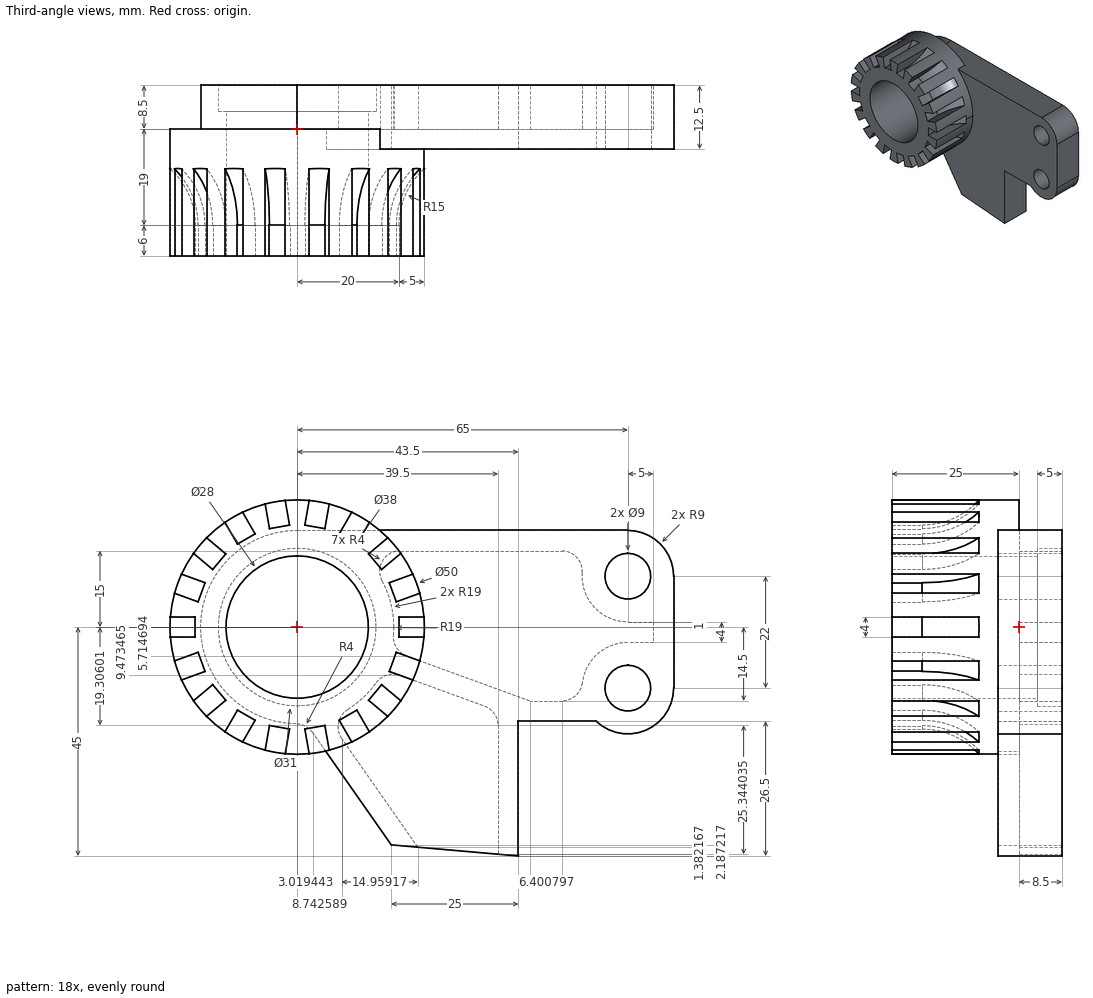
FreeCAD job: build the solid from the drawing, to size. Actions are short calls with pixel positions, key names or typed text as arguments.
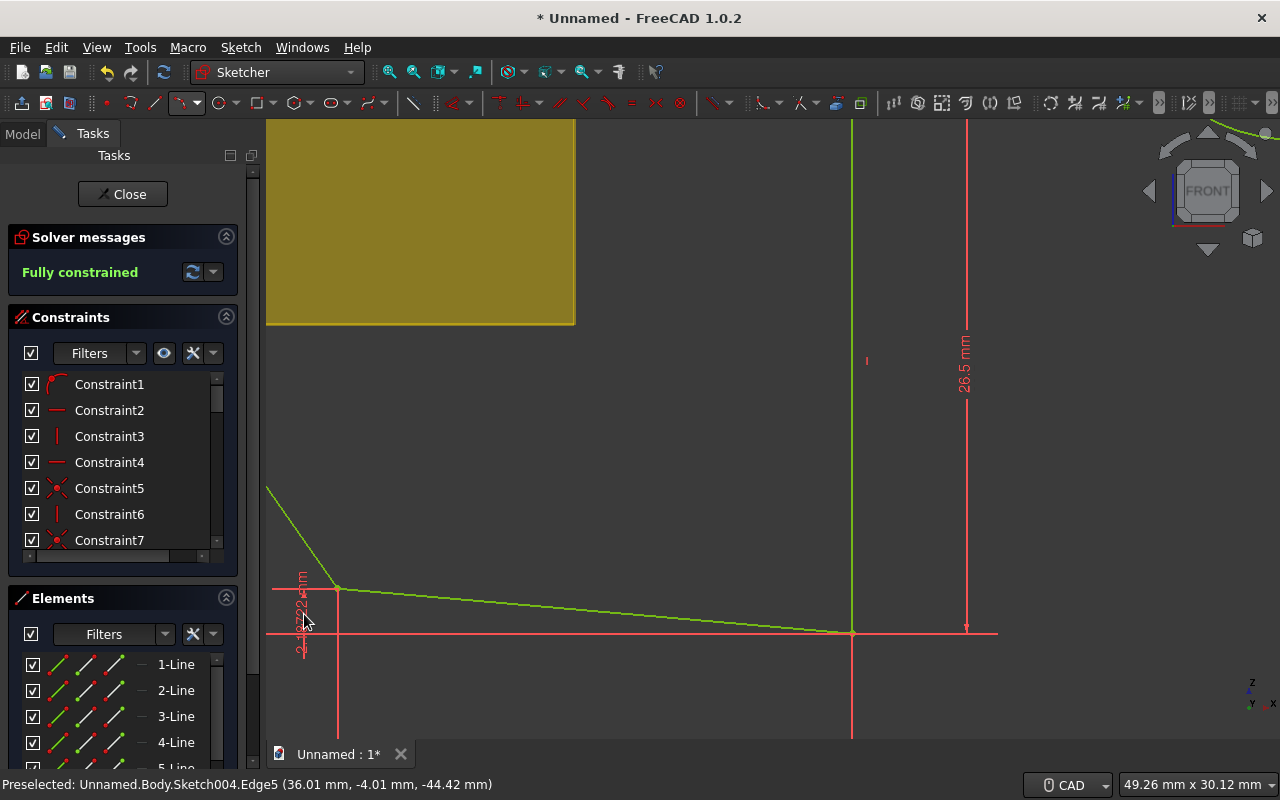
click(123, 194)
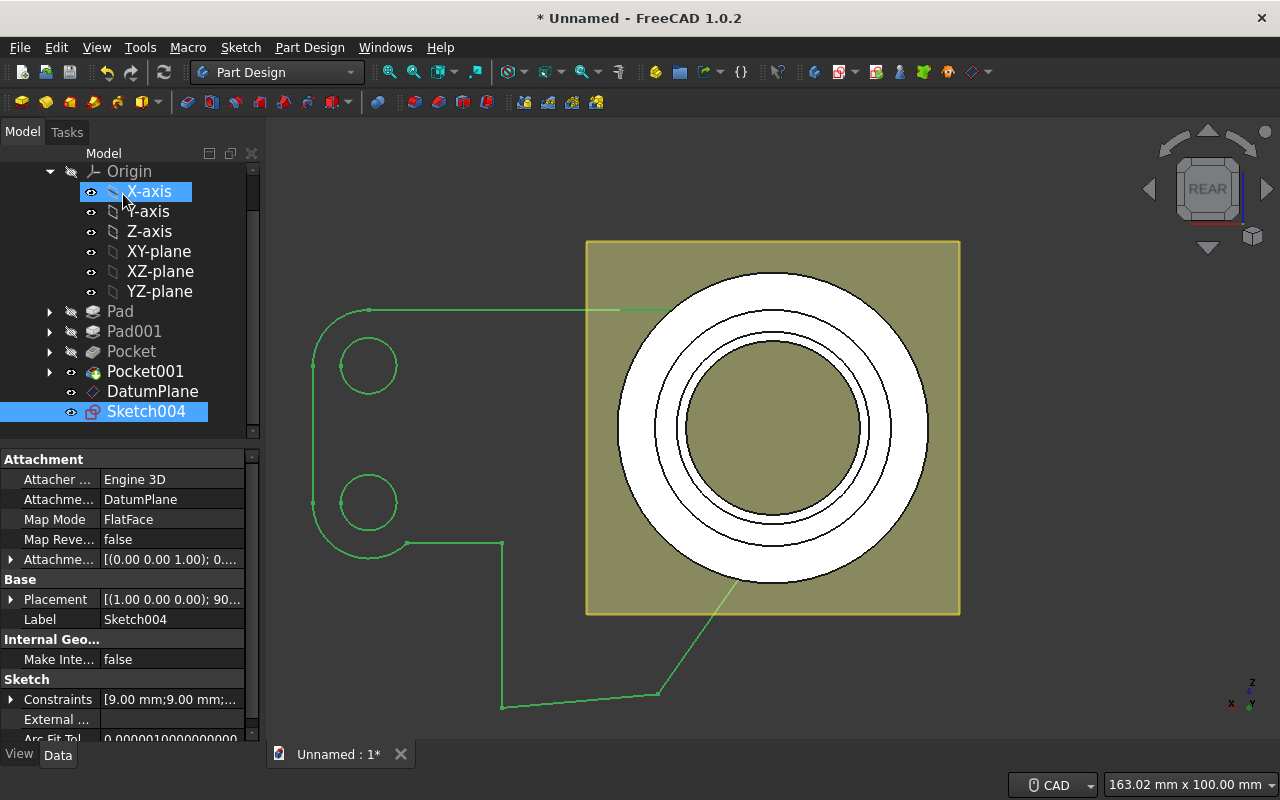
click(22, 102)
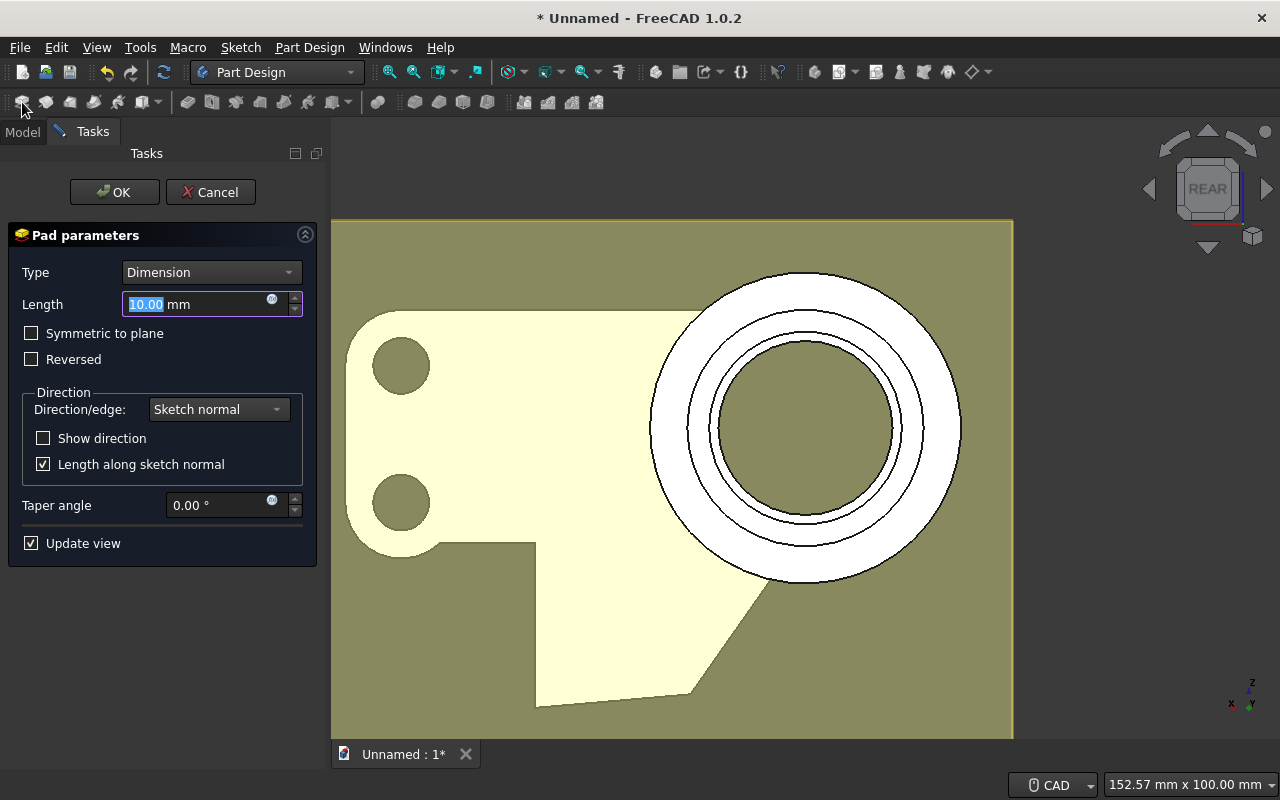
text(12.5)
key(Tab)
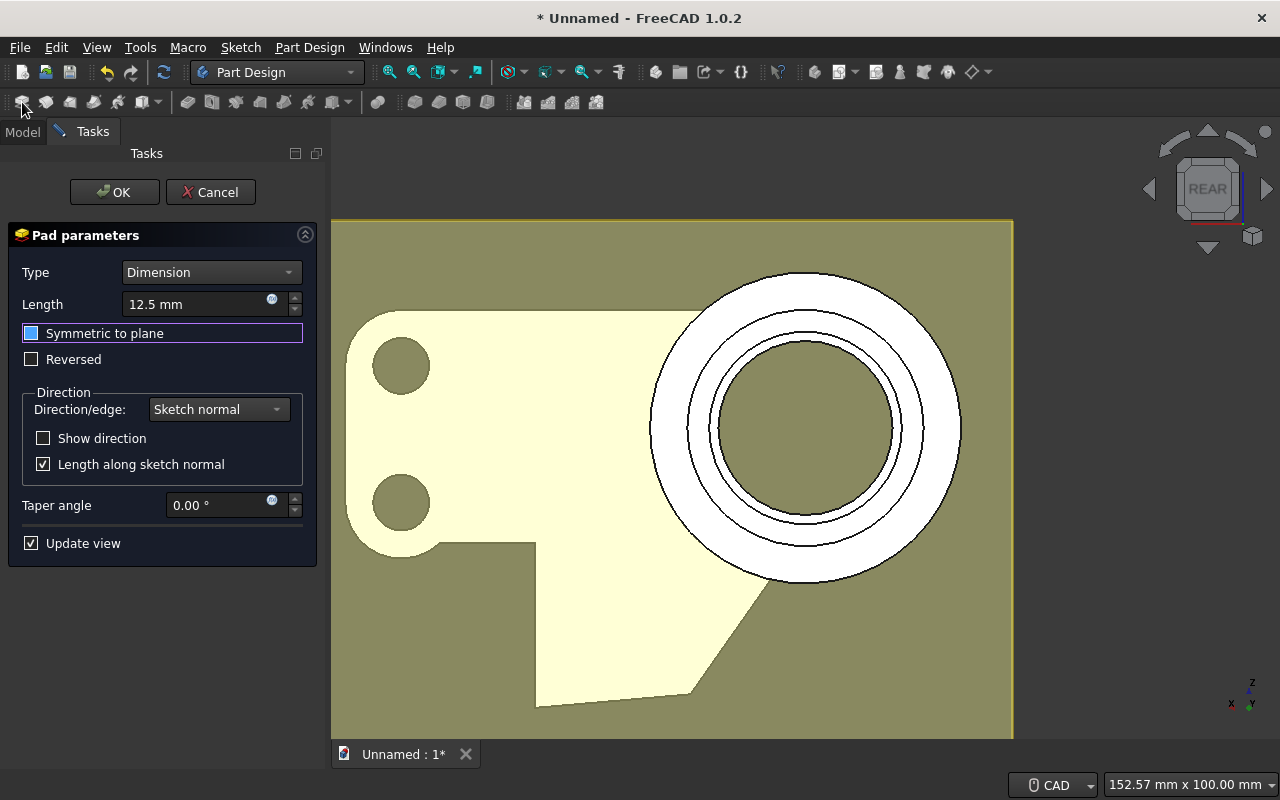
click(30, 359)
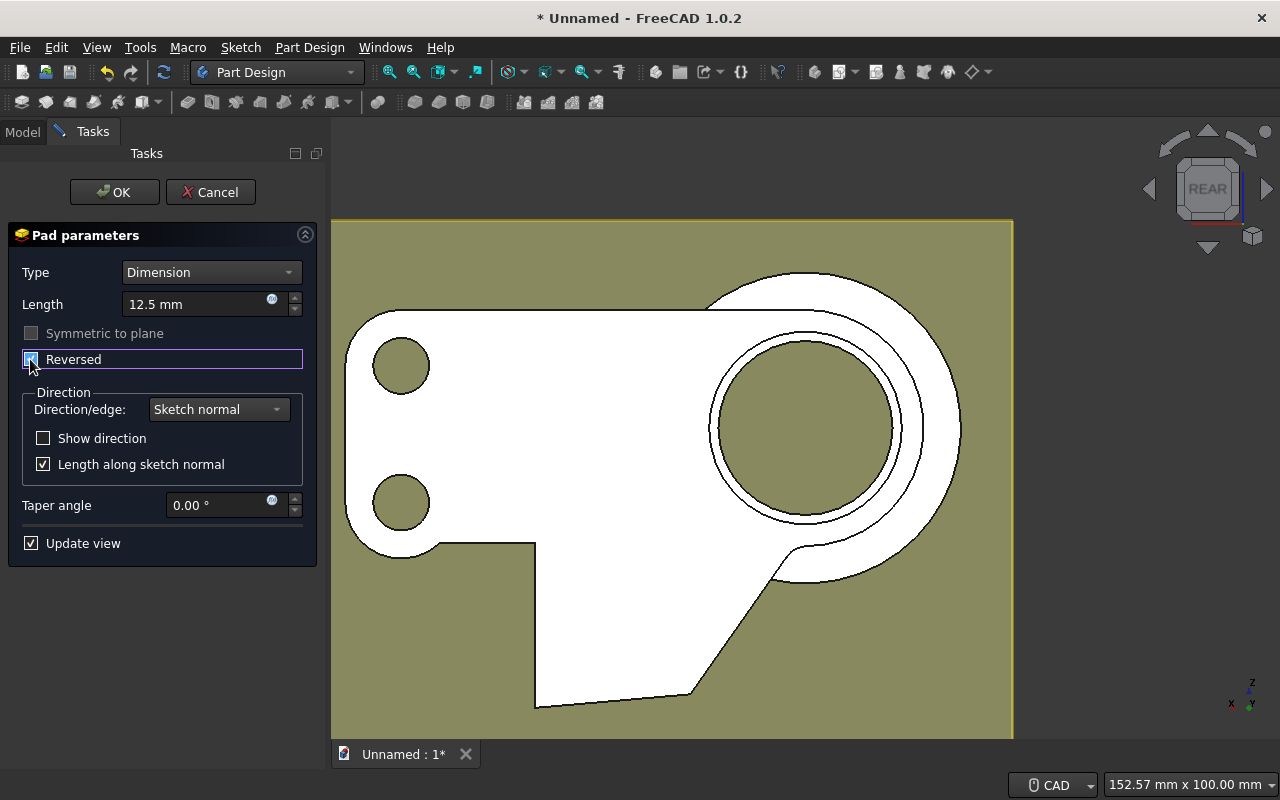
click(115, 192)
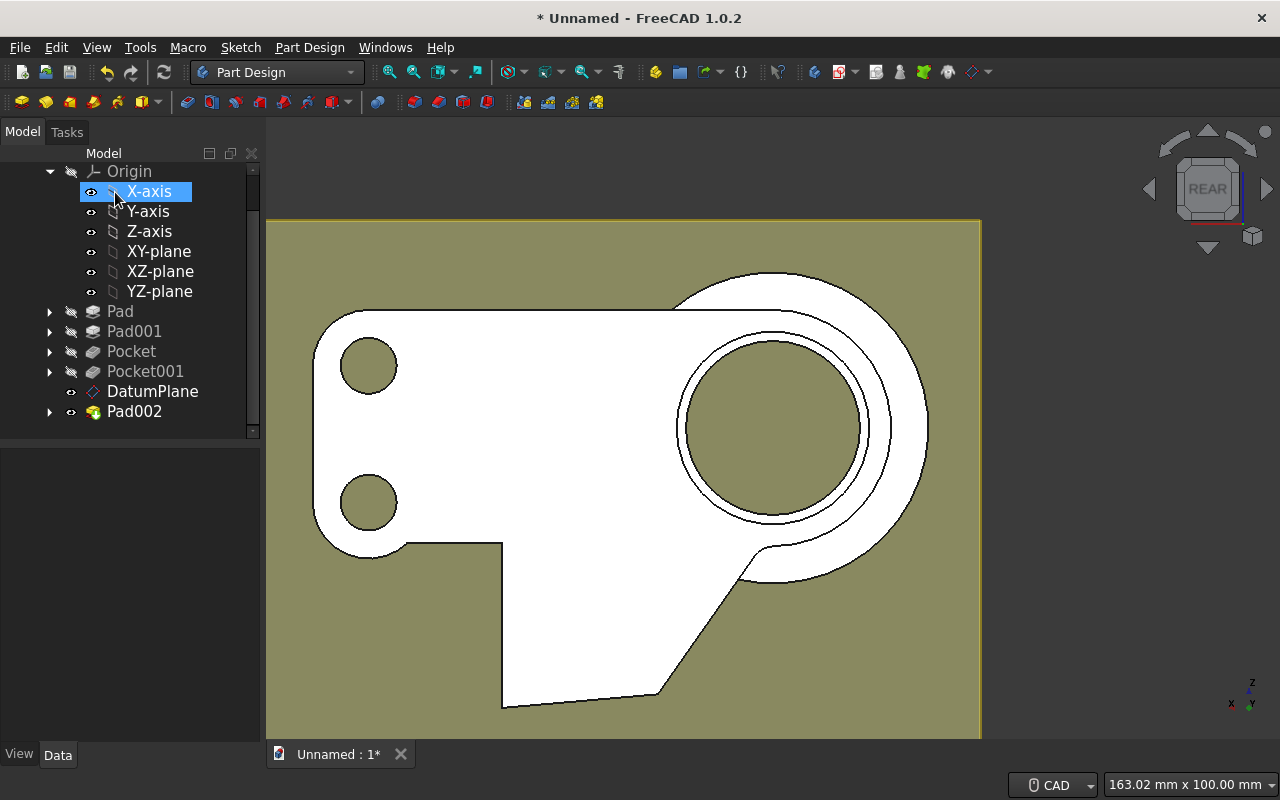
click(116, 392)
key(space)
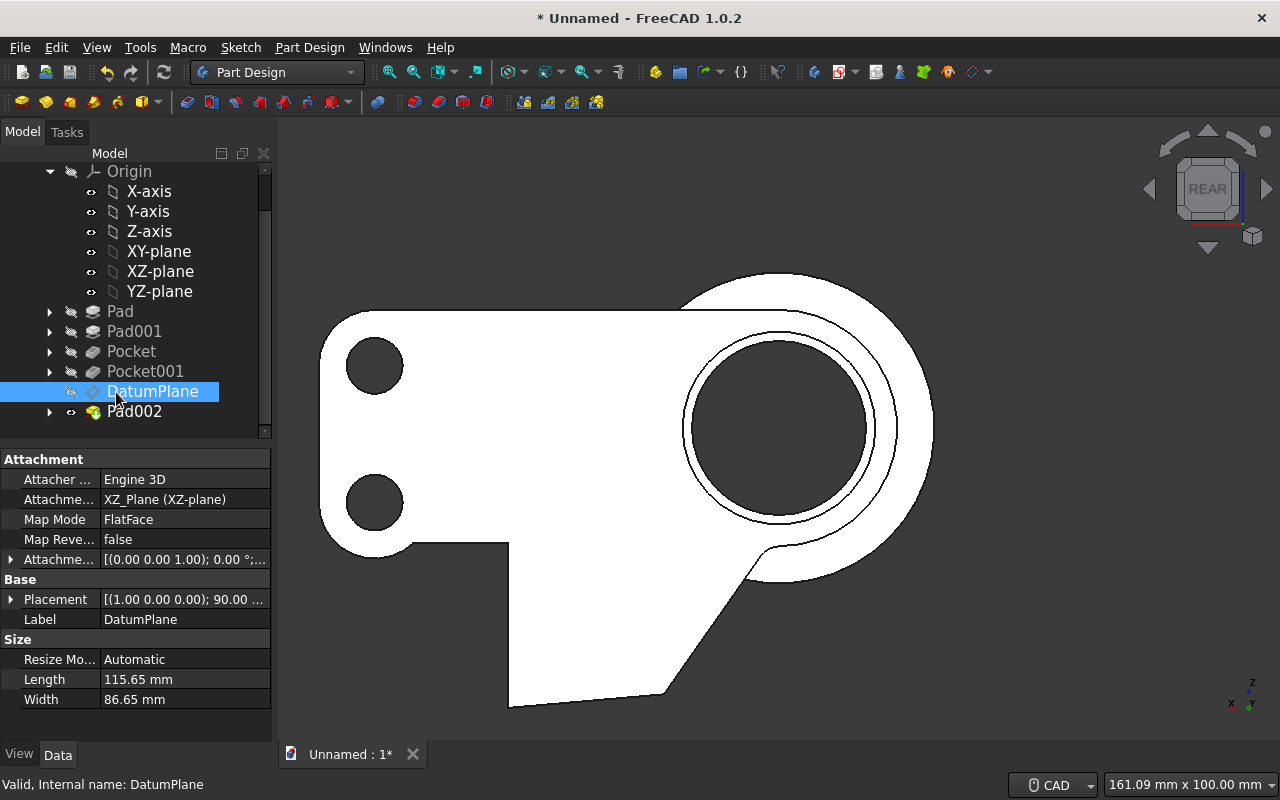
click(318, 699)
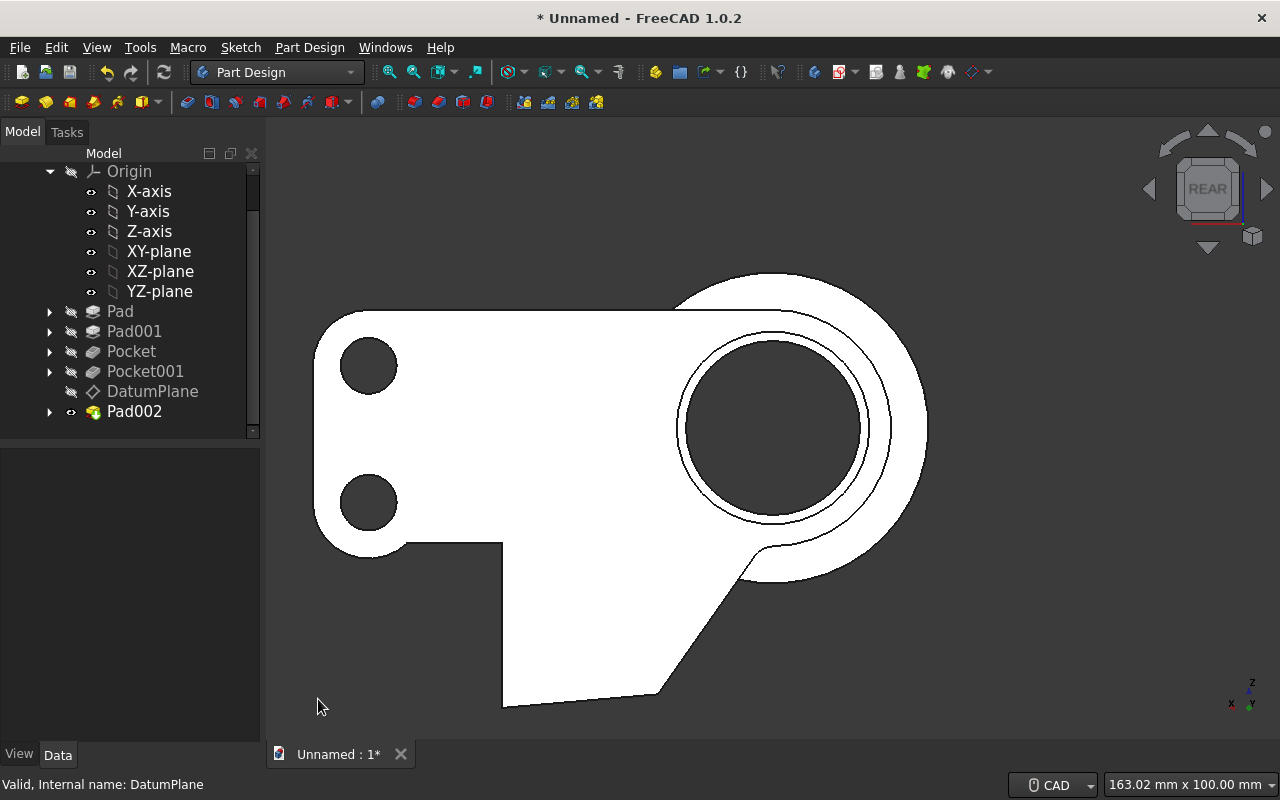
click(840, 72)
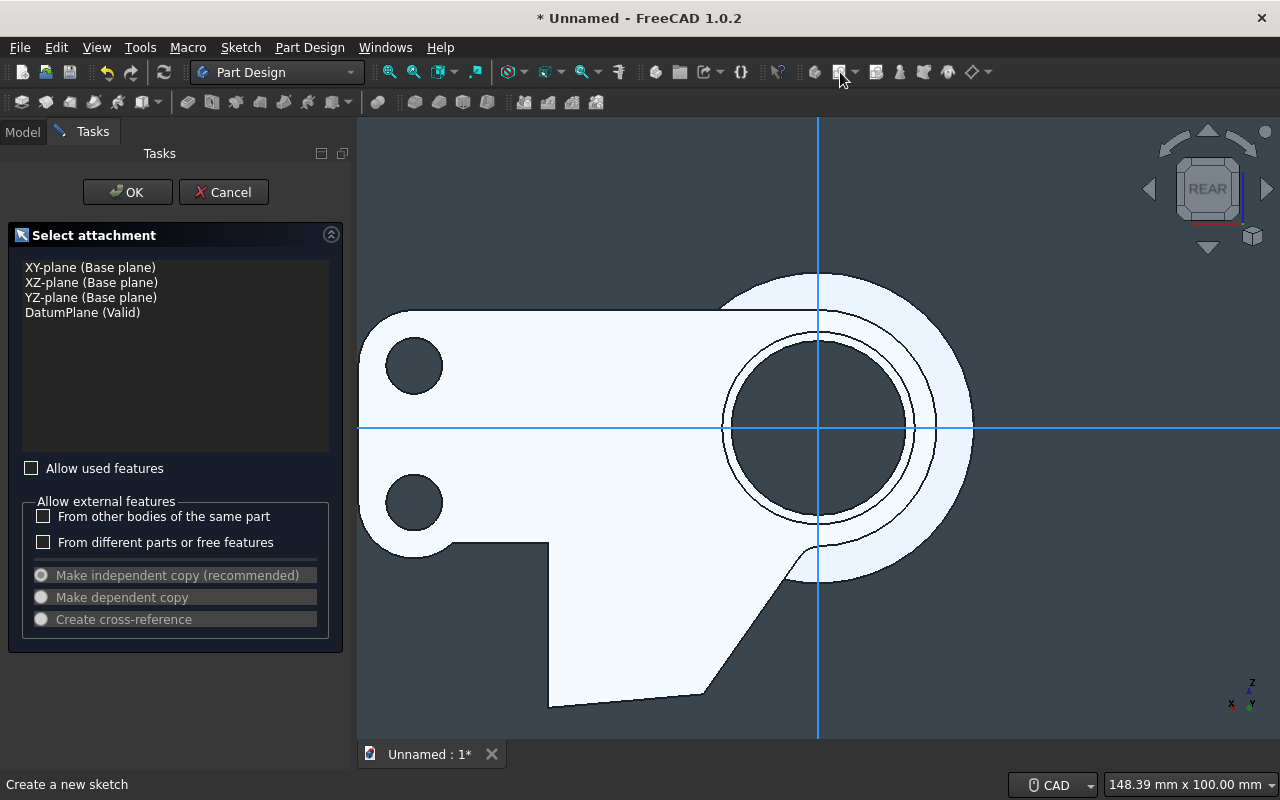
click(82, 282)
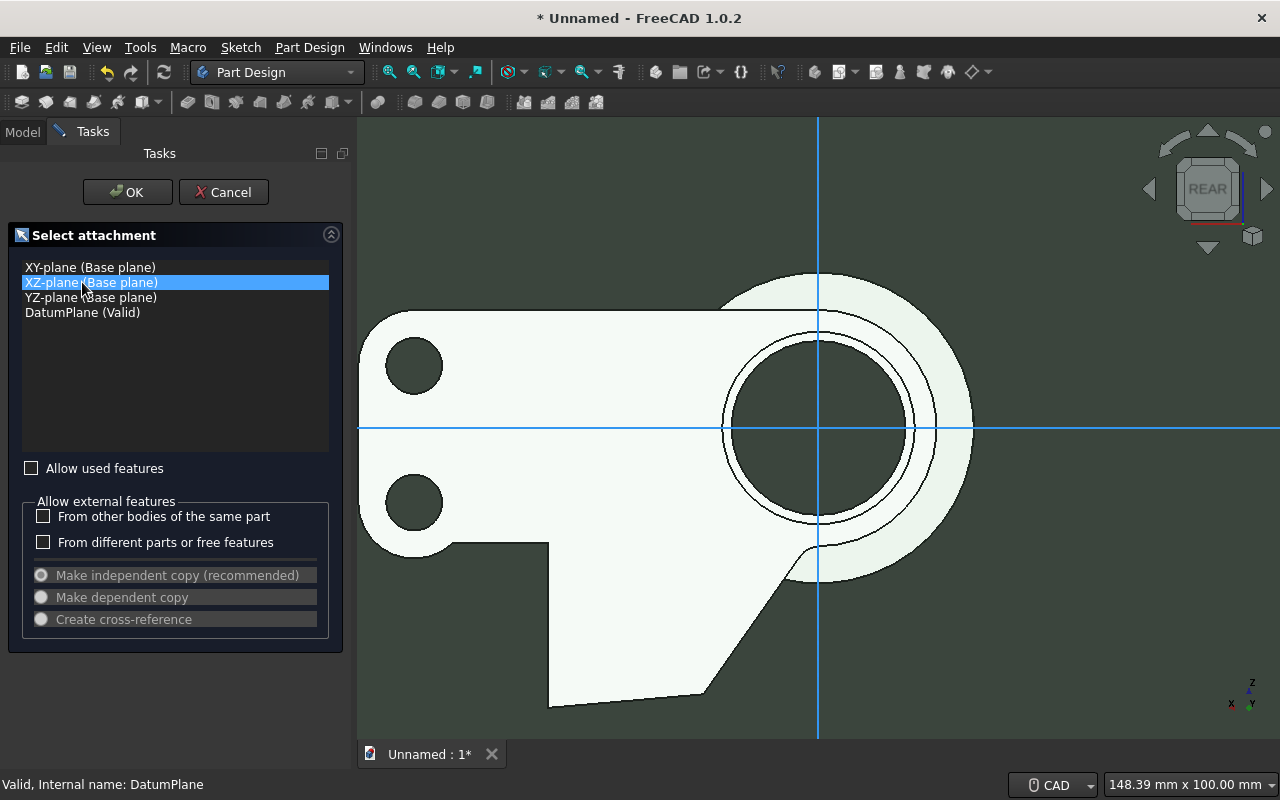
click(128, 192)